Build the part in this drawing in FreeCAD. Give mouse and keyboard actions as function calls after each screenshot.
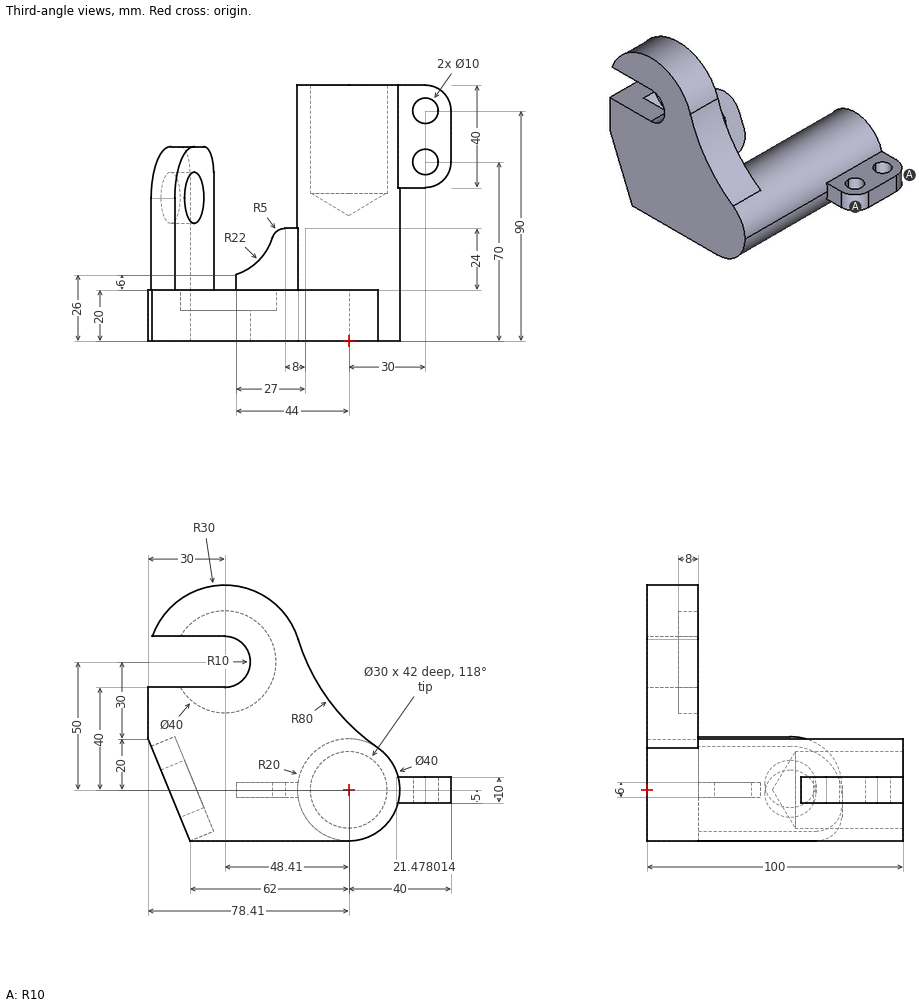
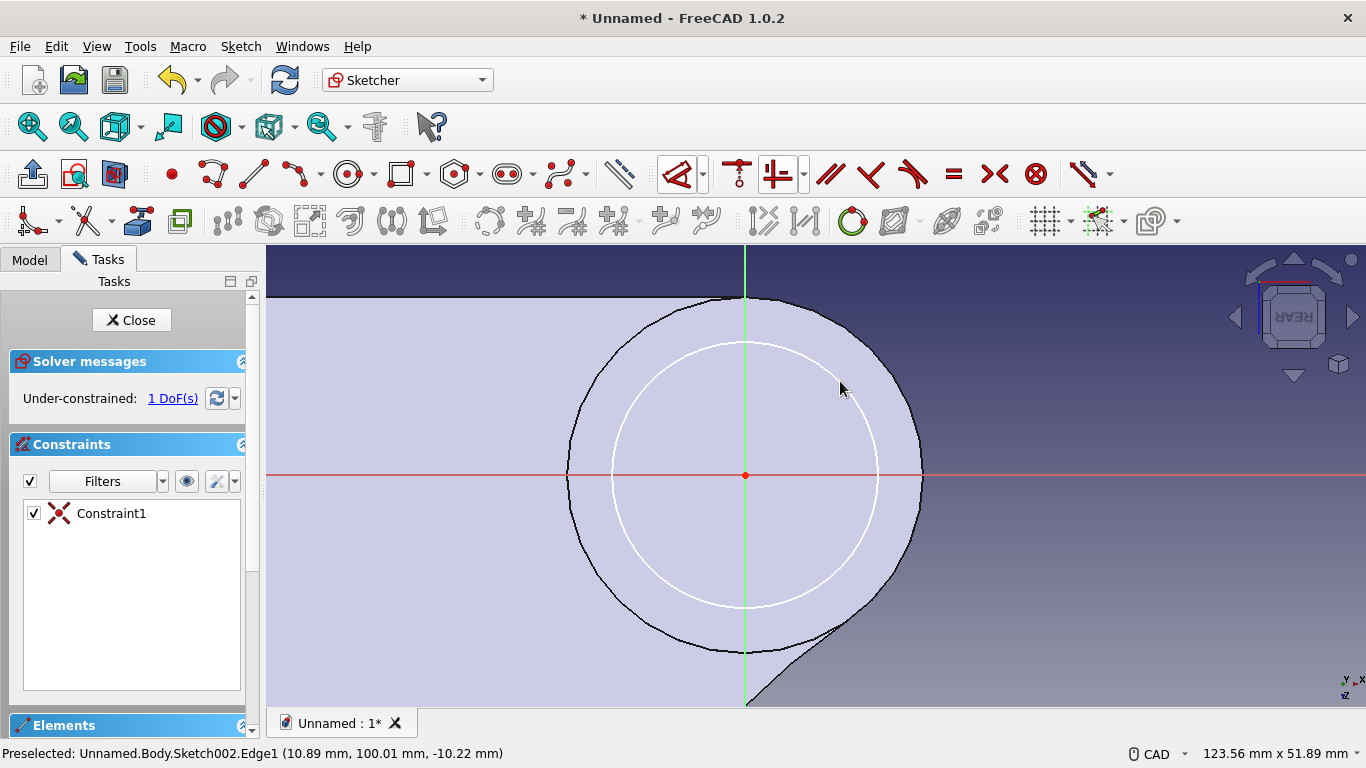
key(d)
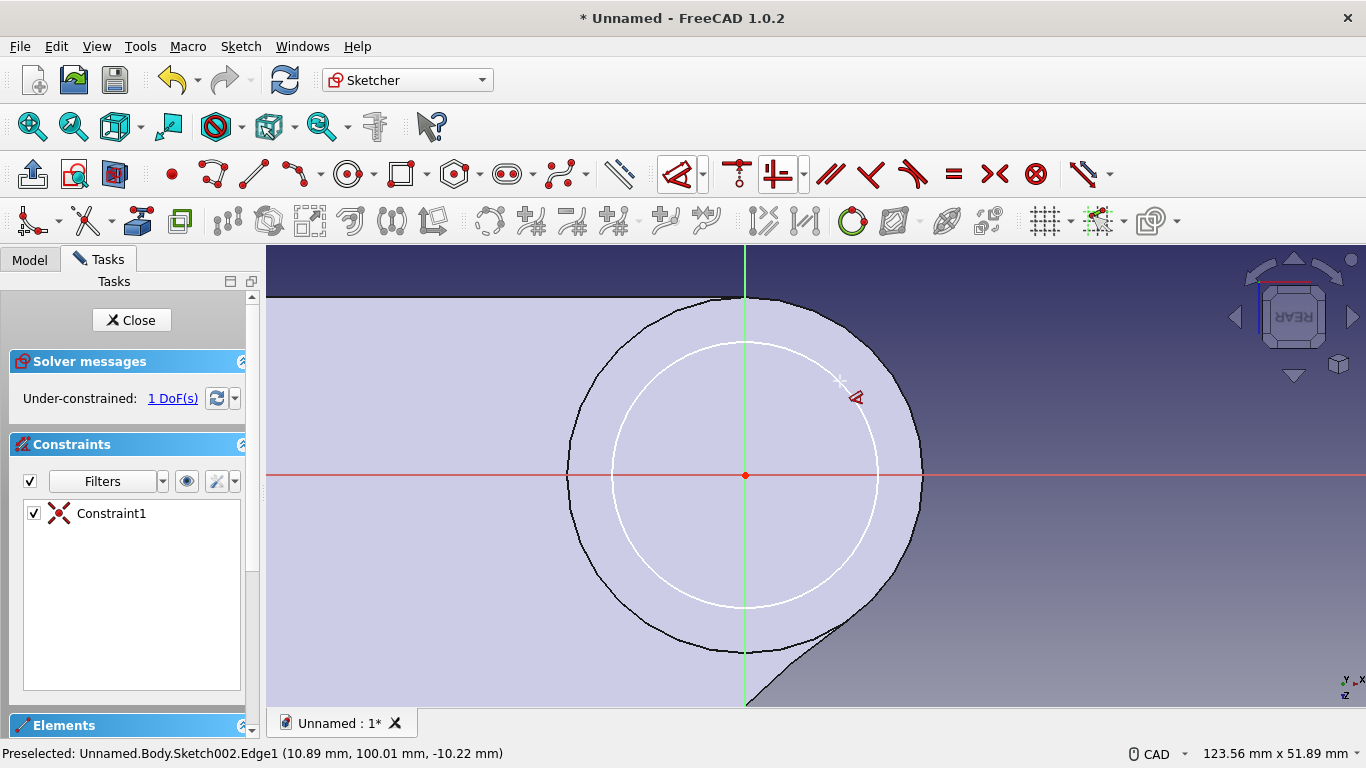
click(839, 381)
click(862, 358)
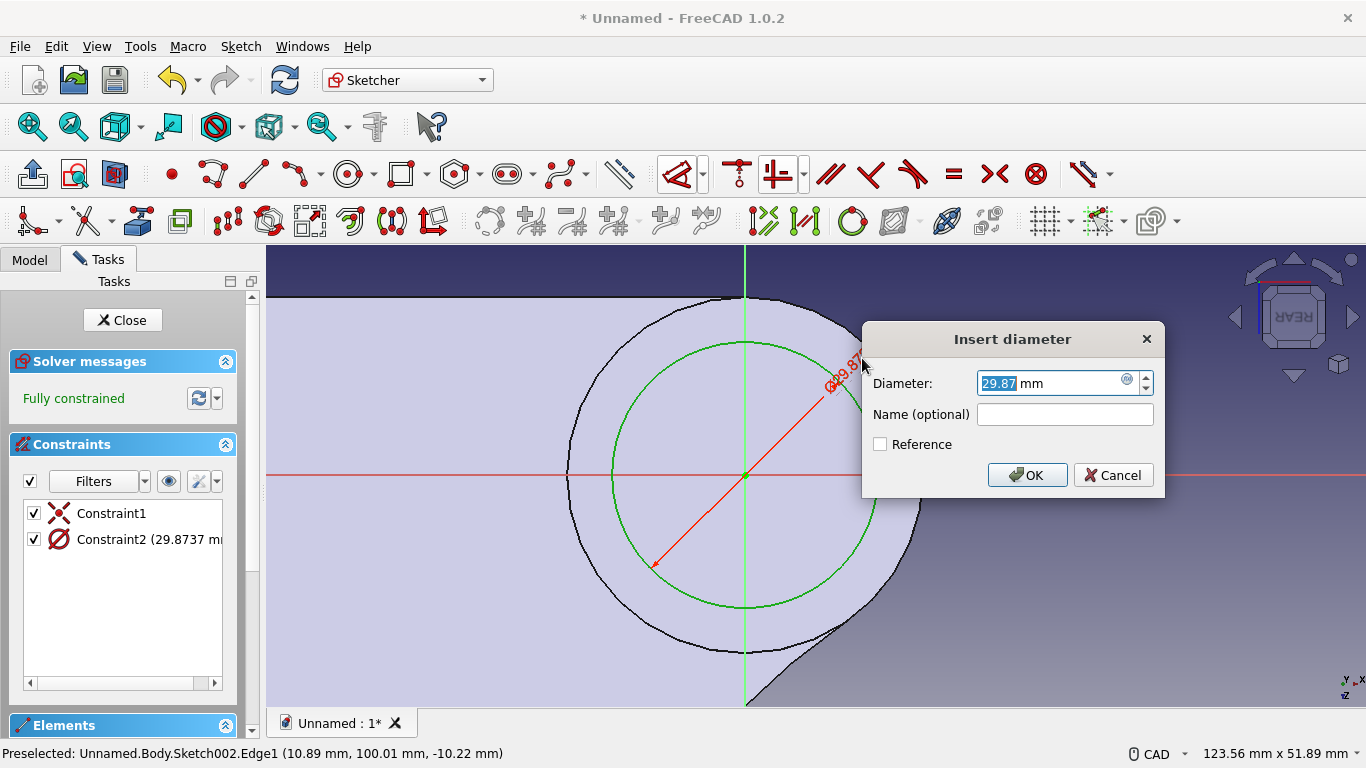
text(30)
key(Return)
key(Escape)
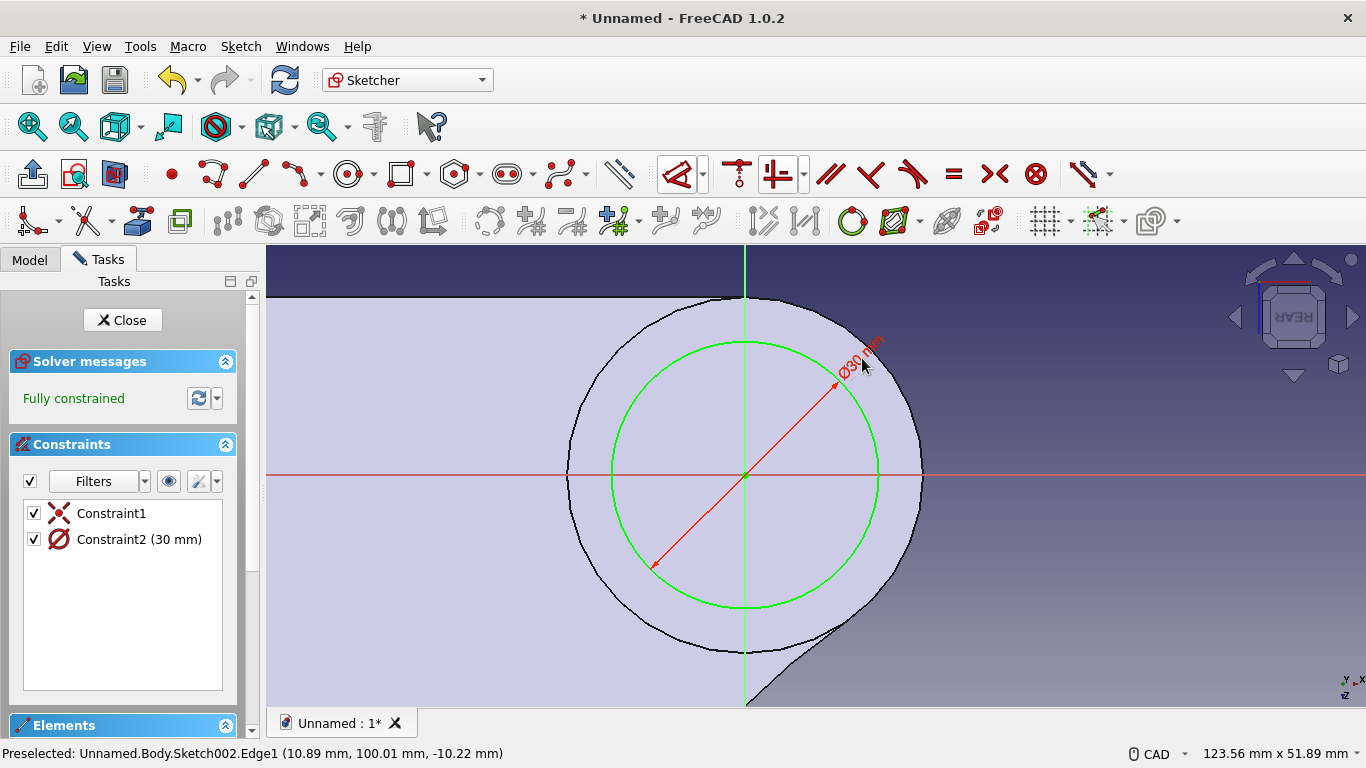
click(123, 320)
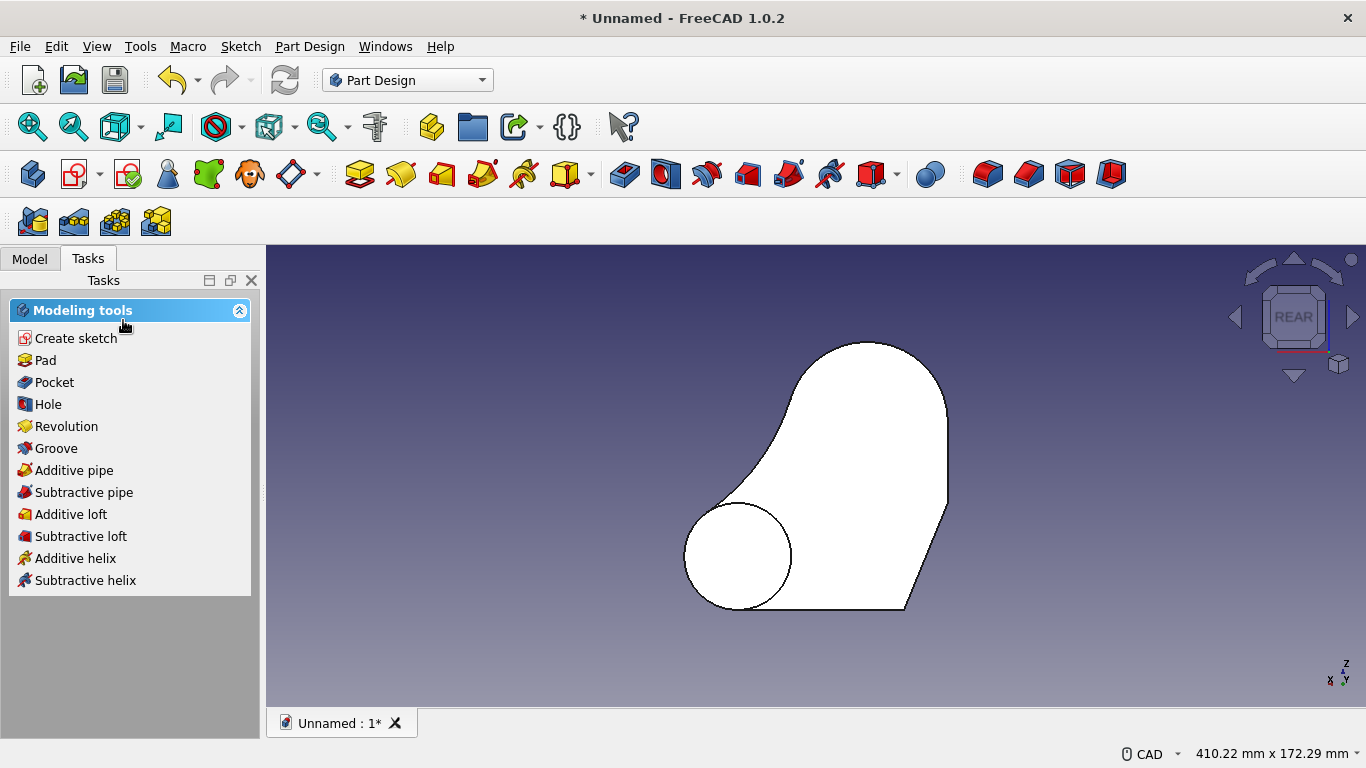
click(666, 174)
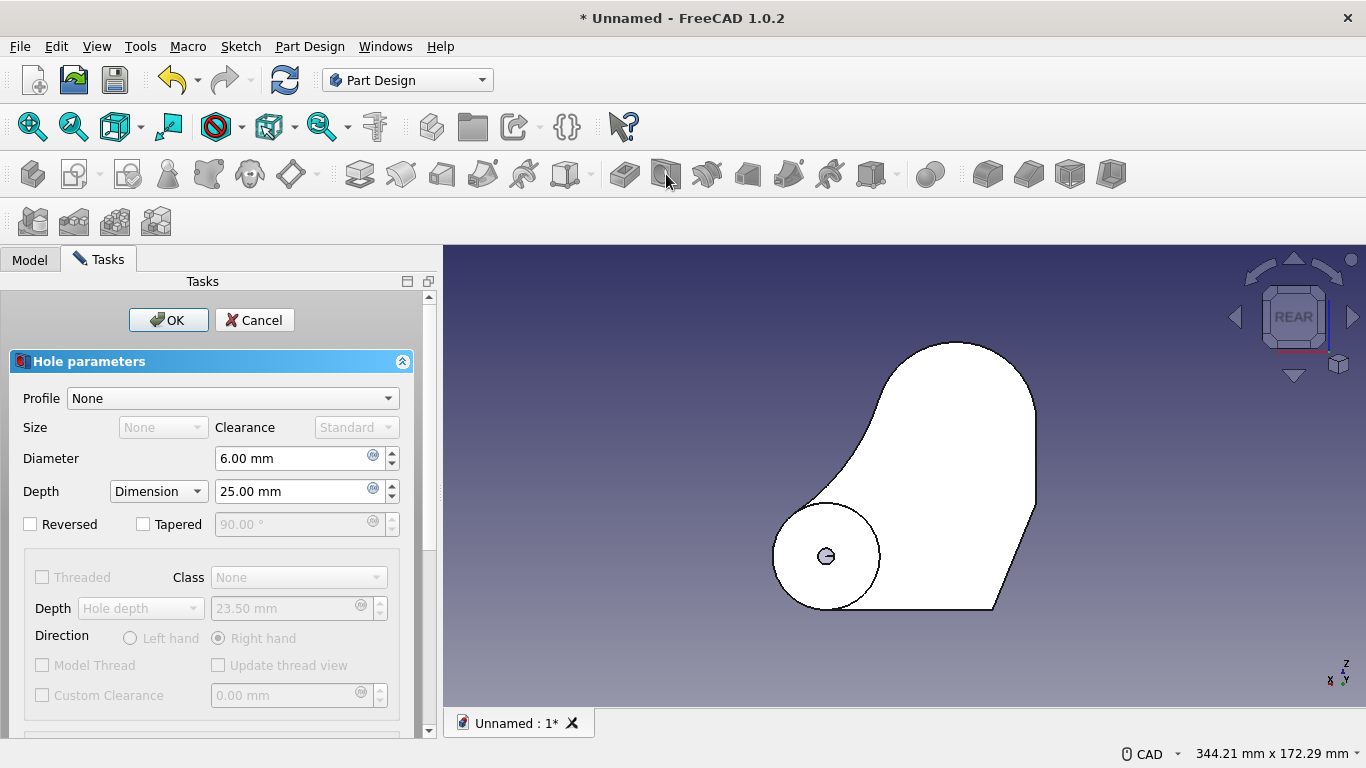
triple_click(300, 458)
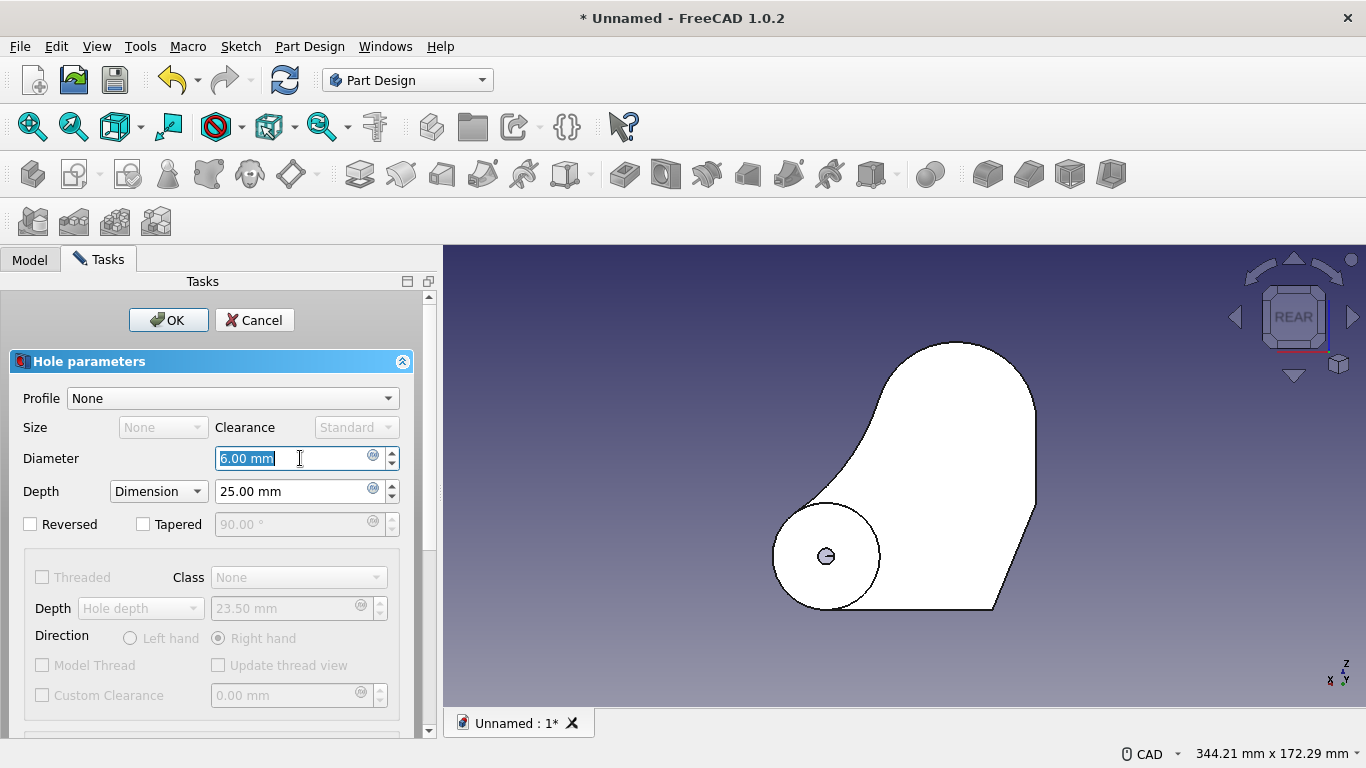
text(30)
key(Tab)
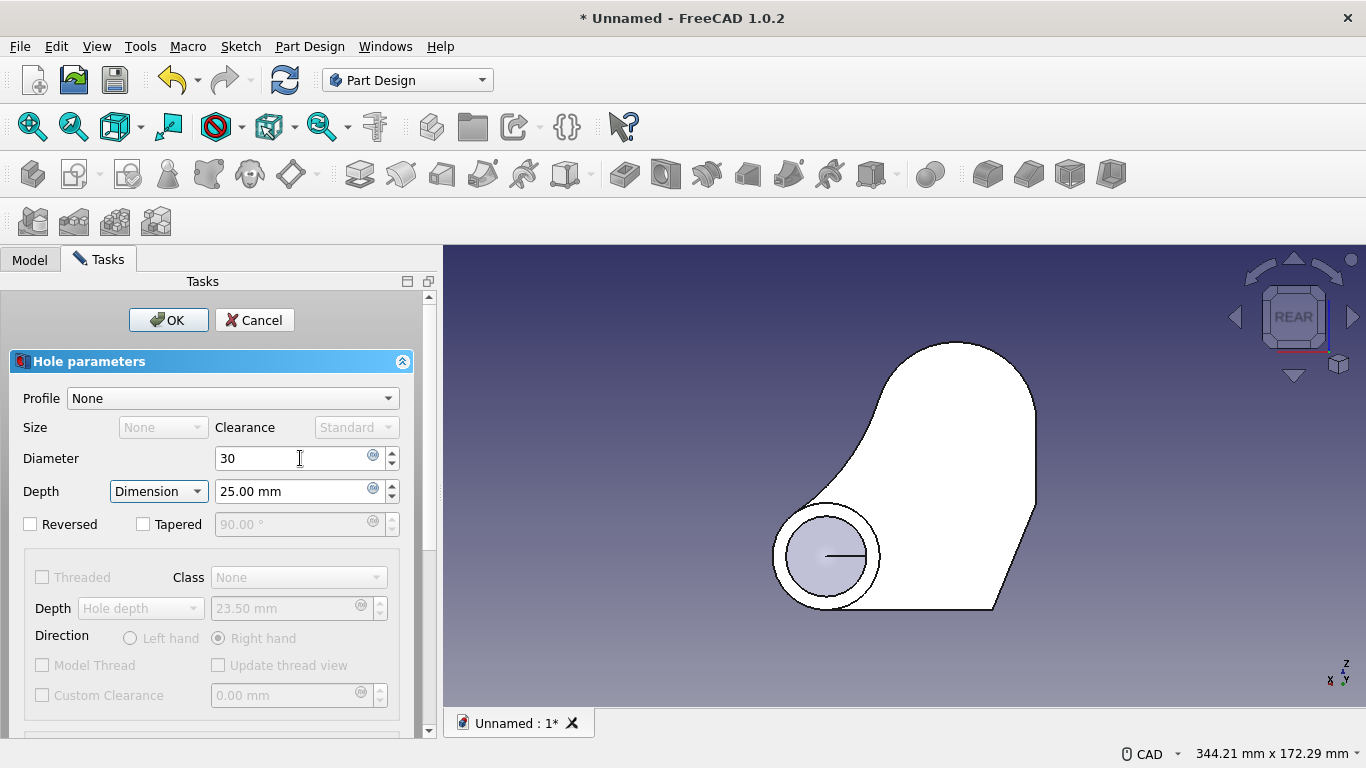
triple_click(300, 492)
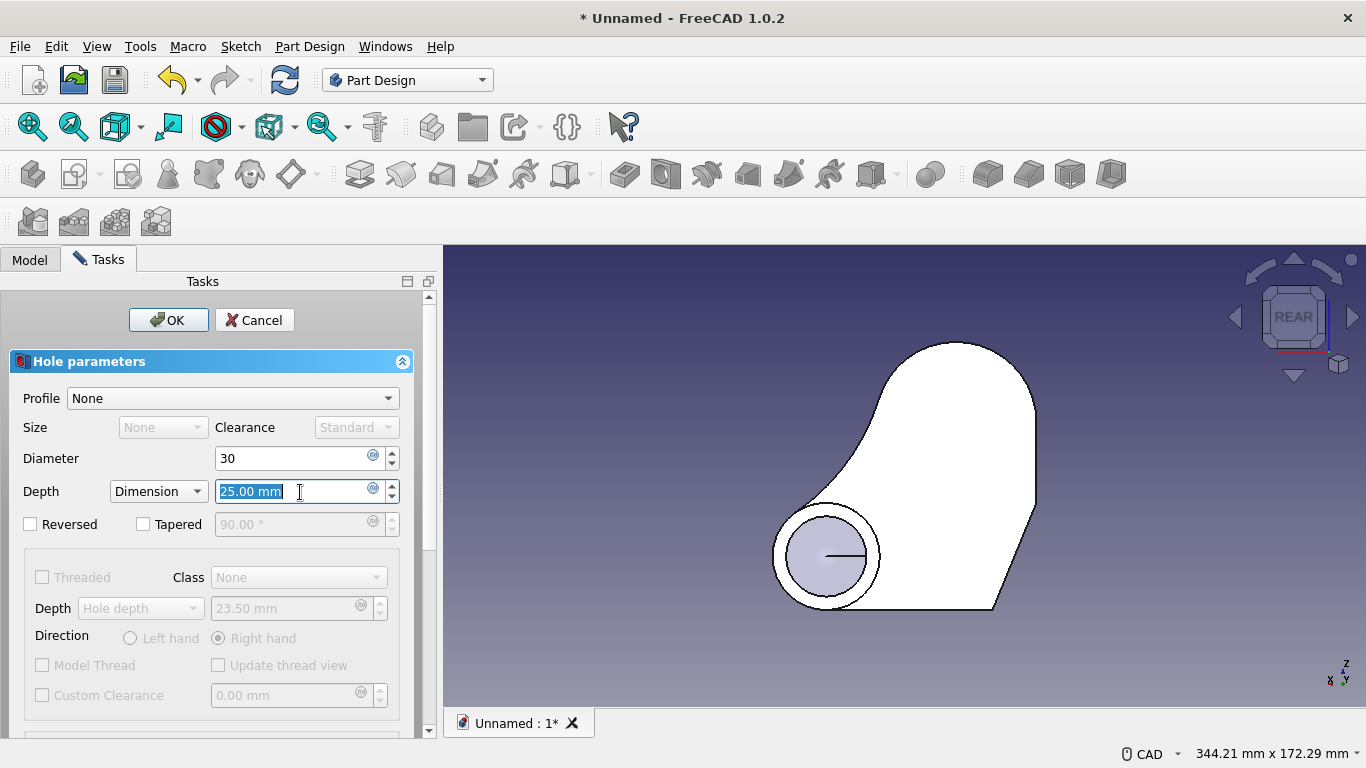
text(42)
key(Tab)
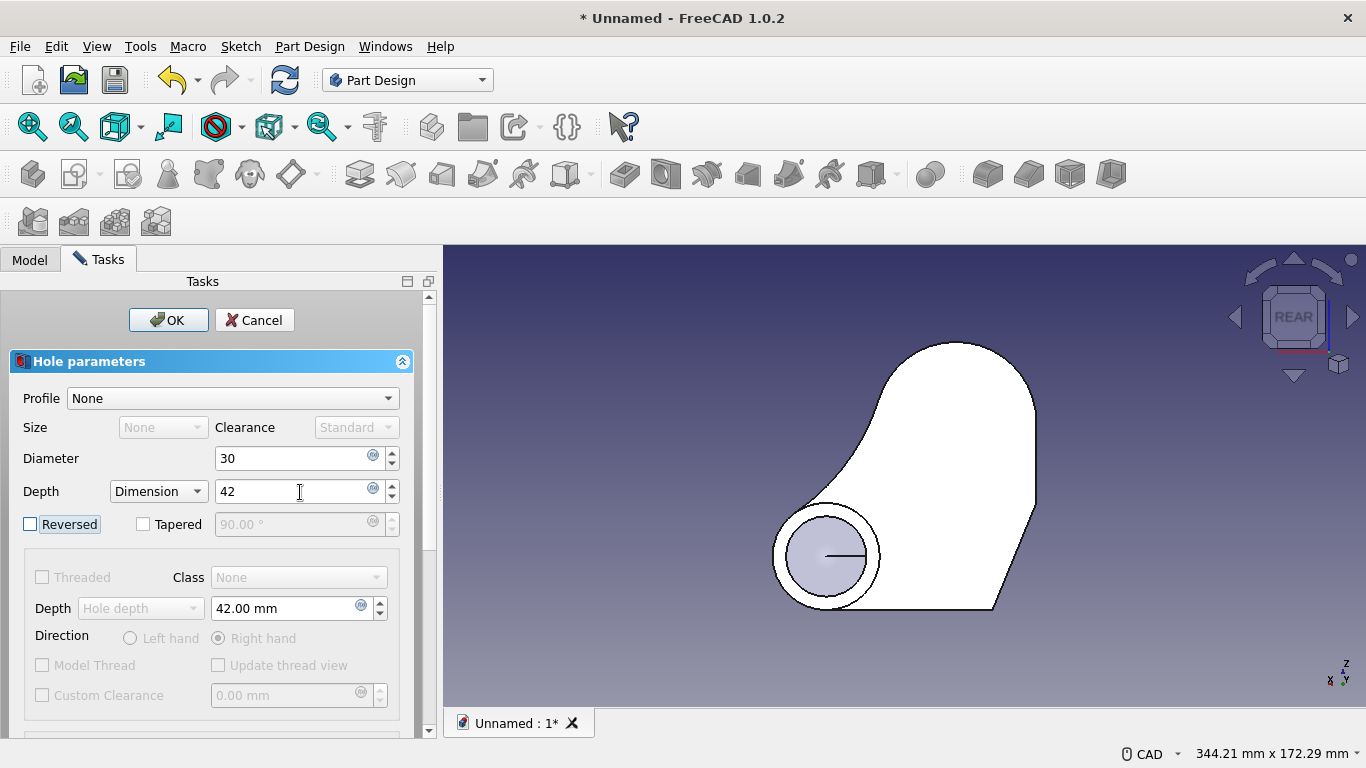
click(169, 320)